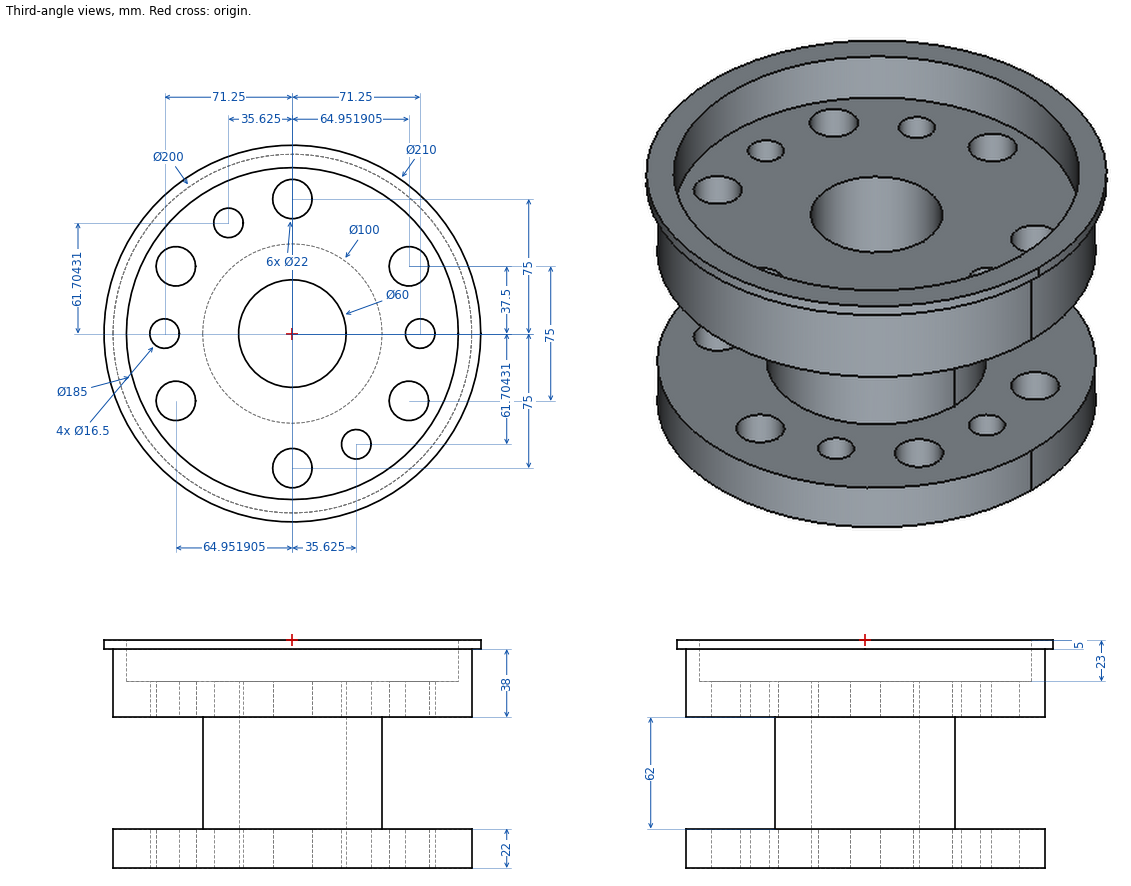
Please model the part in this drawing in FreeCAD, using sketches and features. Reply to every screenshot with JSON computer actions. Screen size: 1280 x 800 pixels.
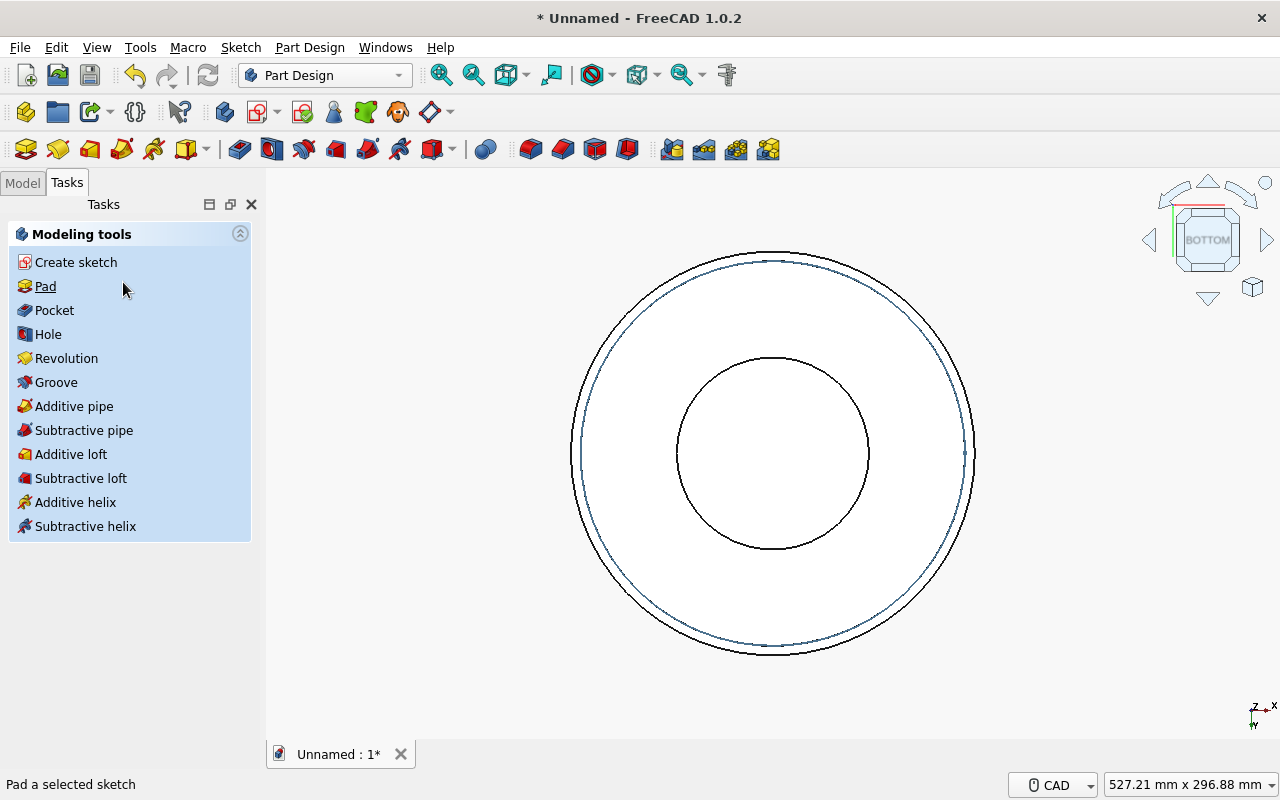
{"action": "left_click", "coordinate": [26, 150]}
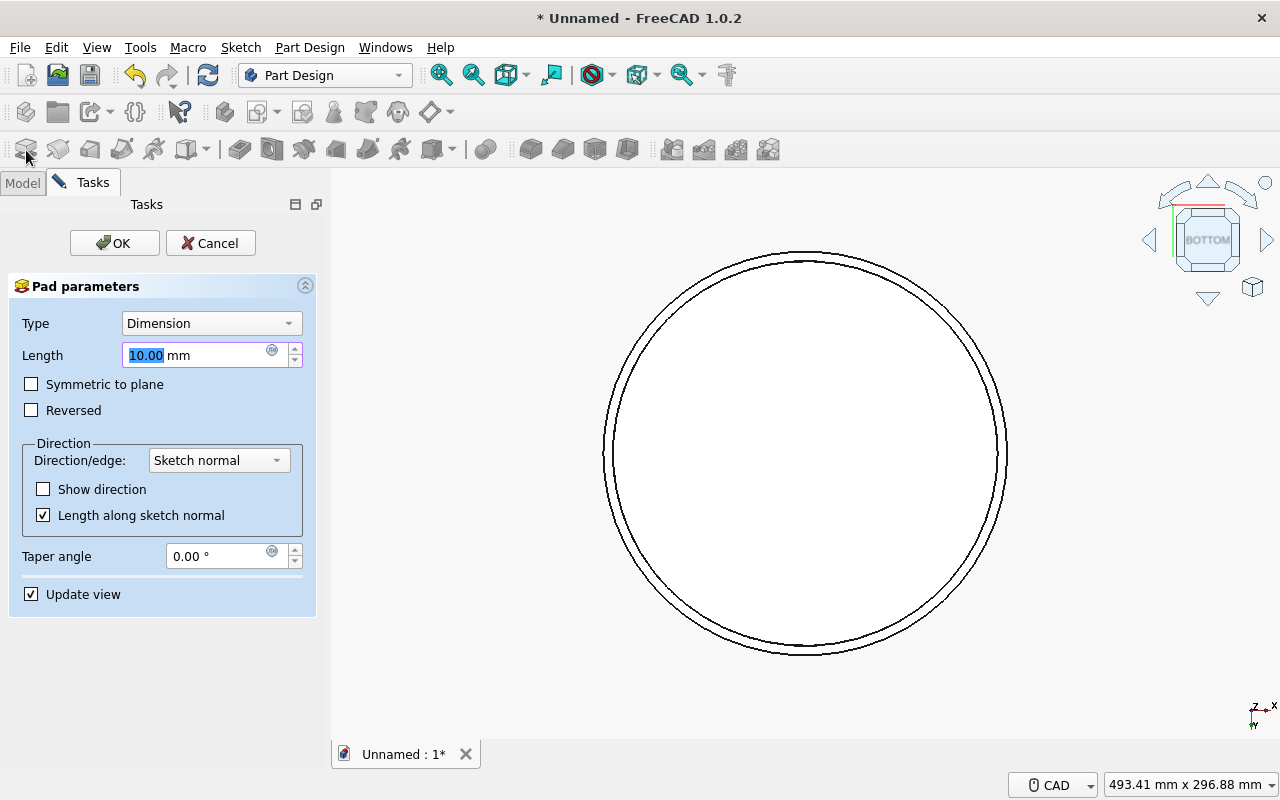
{"action": "type", "text": "22"}
{"action": "key", "text": "Tab"}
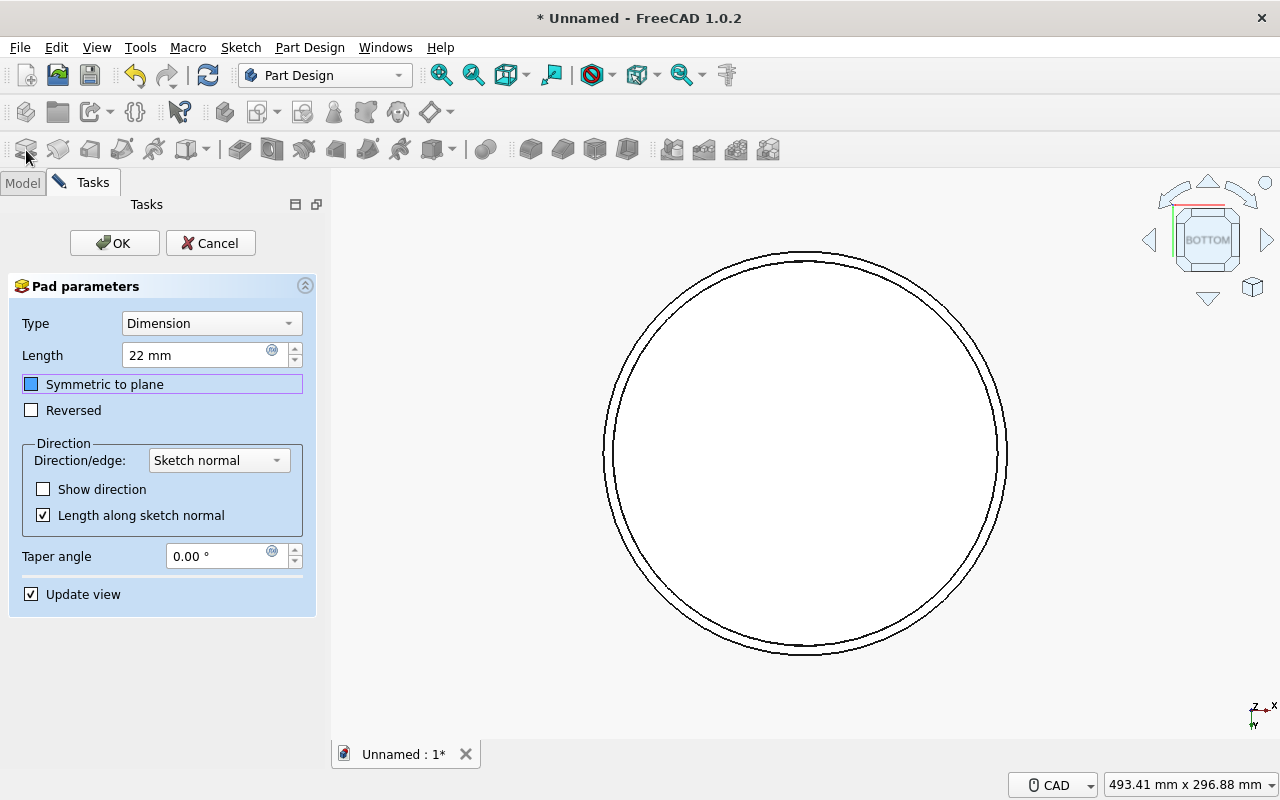
{"action": "left_click", "coordinate": [115, 243]}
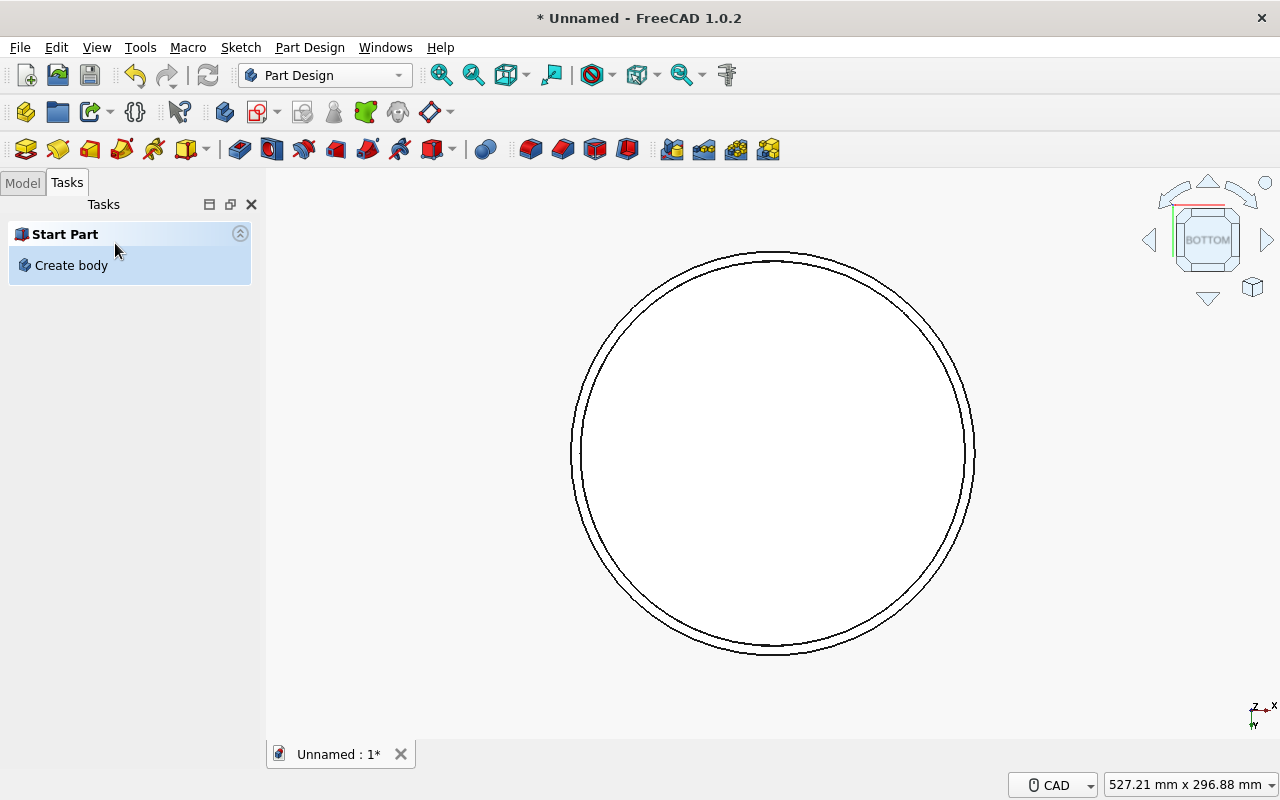
{"action": "key", "text": "0"}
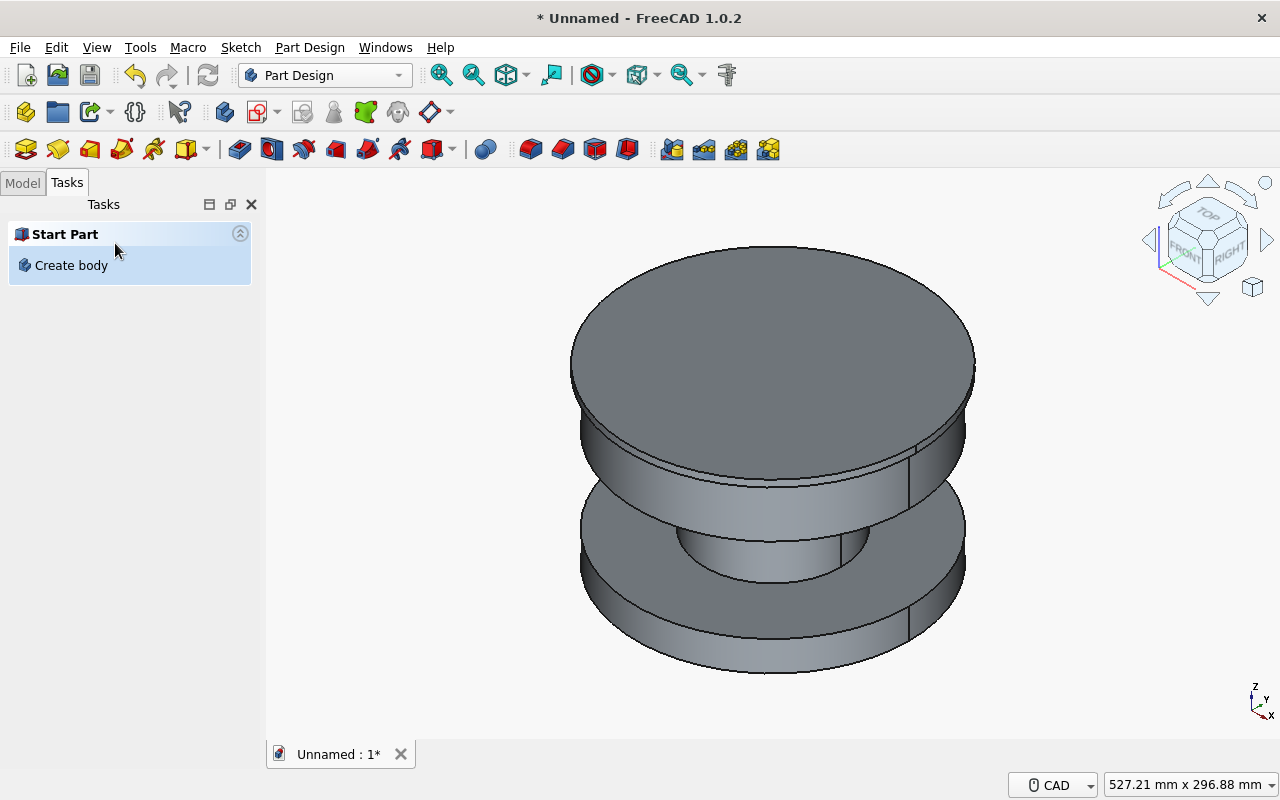
{"action": "left_click", "coordinate": [773, 362]}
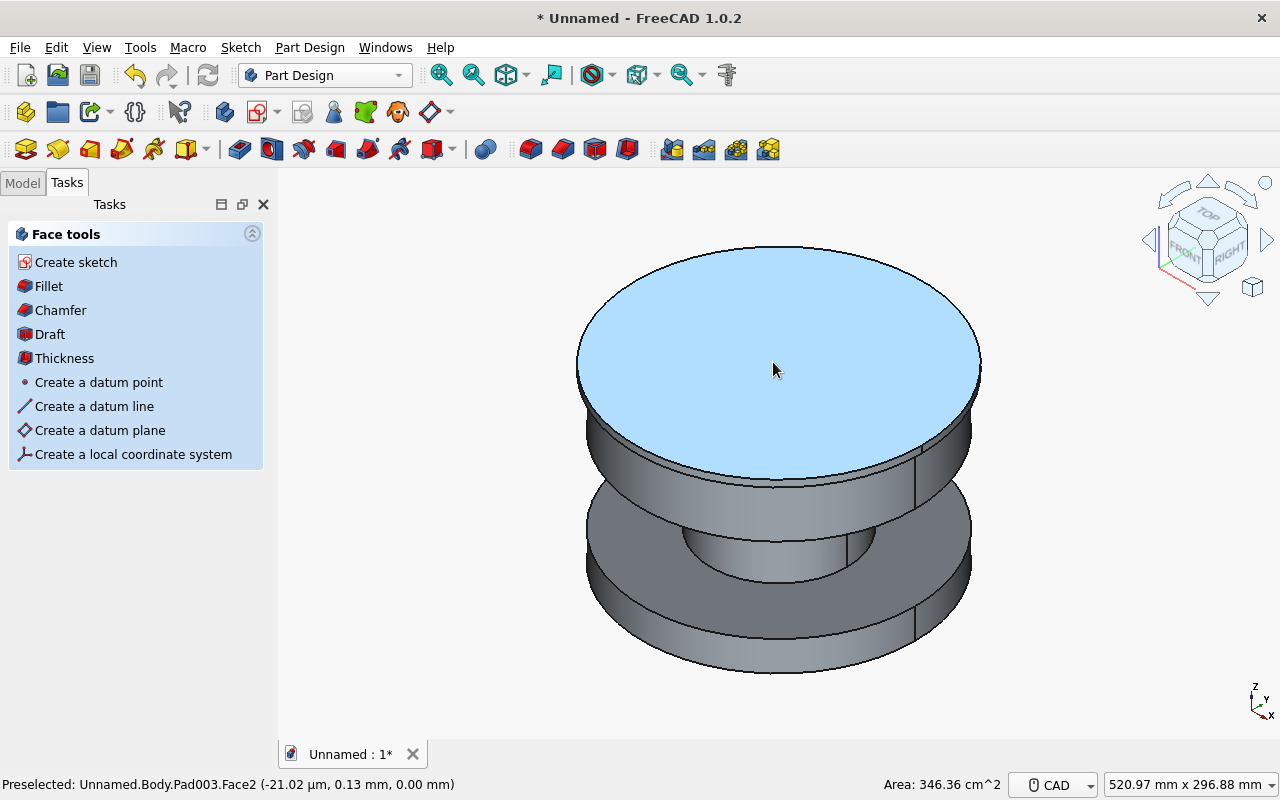
{"action": "left_click", "coordinate": [258, 112]}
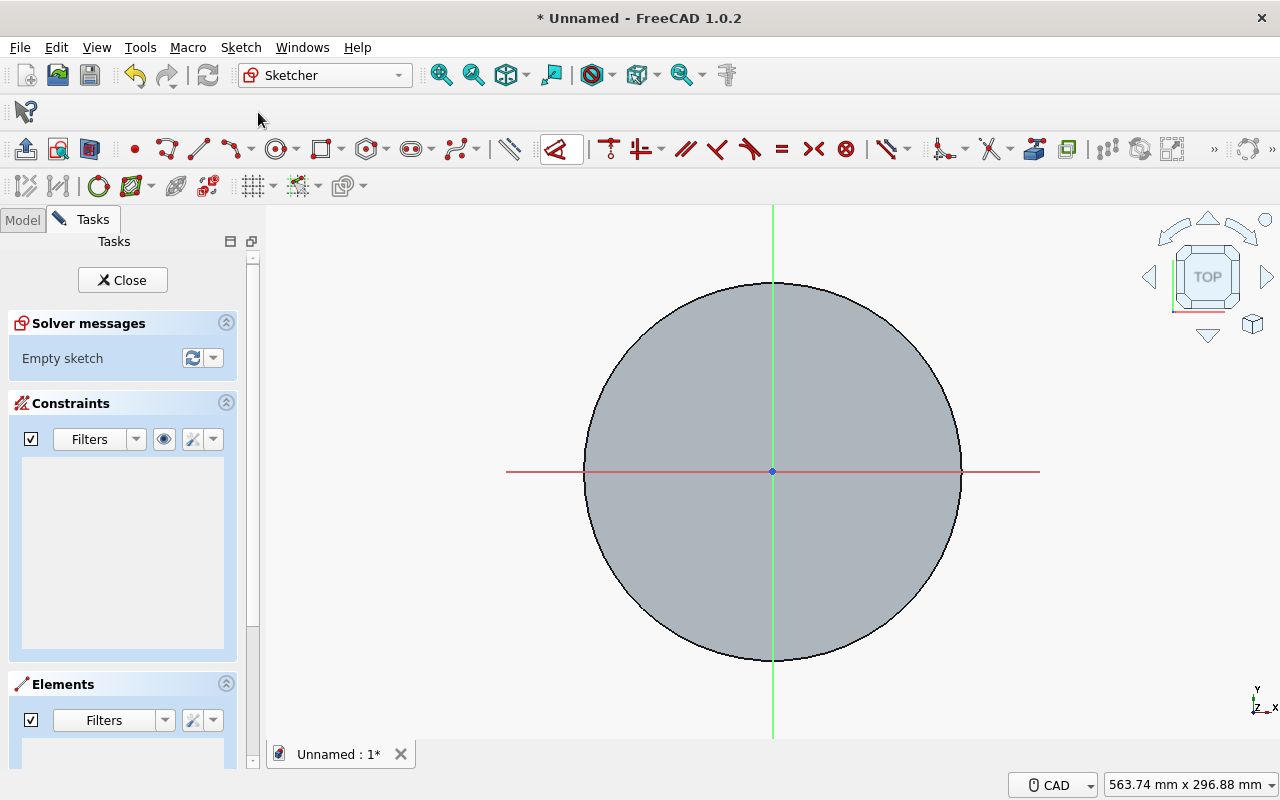
{"action": "left_click", "coordinate": [276, 150]}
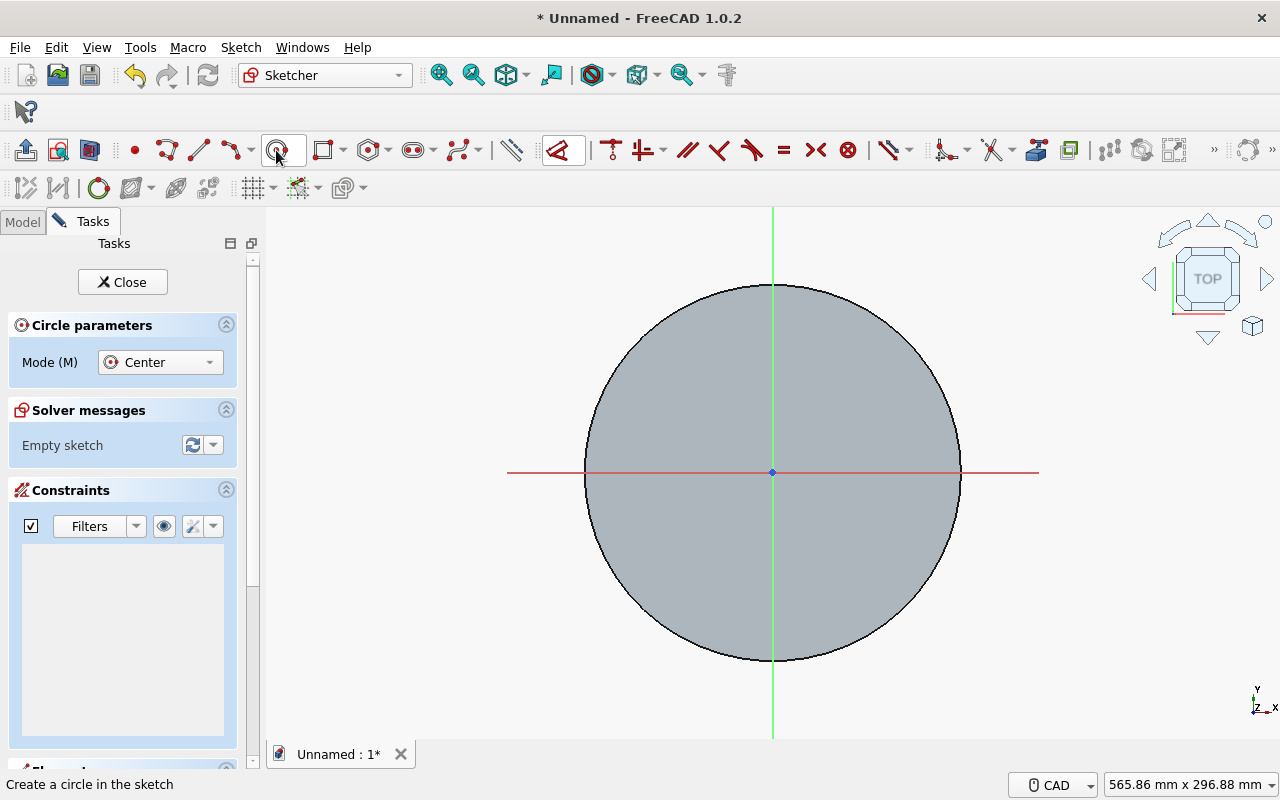
{"action": "left_click", "coordinate": [773, 473]}
{"action": "mouse_move", "coordinate": [890, 356]}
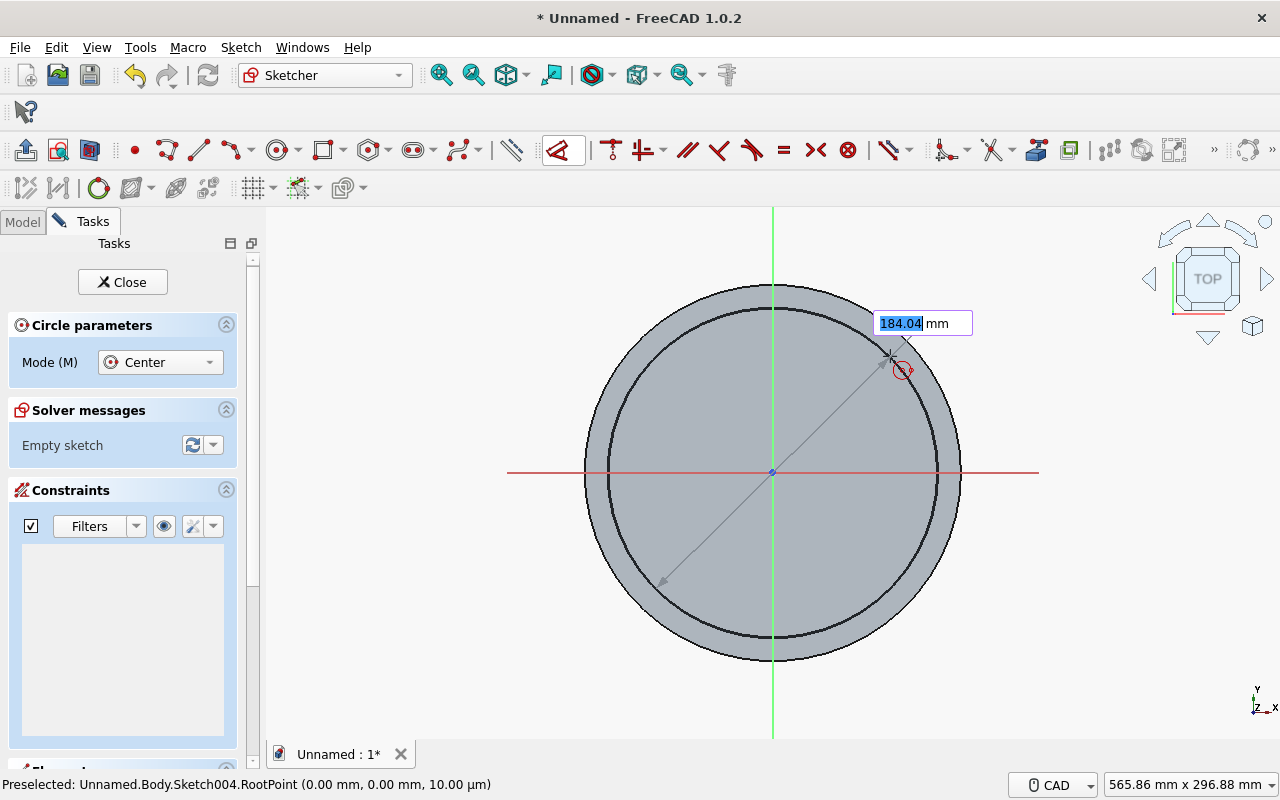
{"action": "type", "text": "185"}
{"action": "key", "text": "Return"}
{"action": "key", "text": "Escape"}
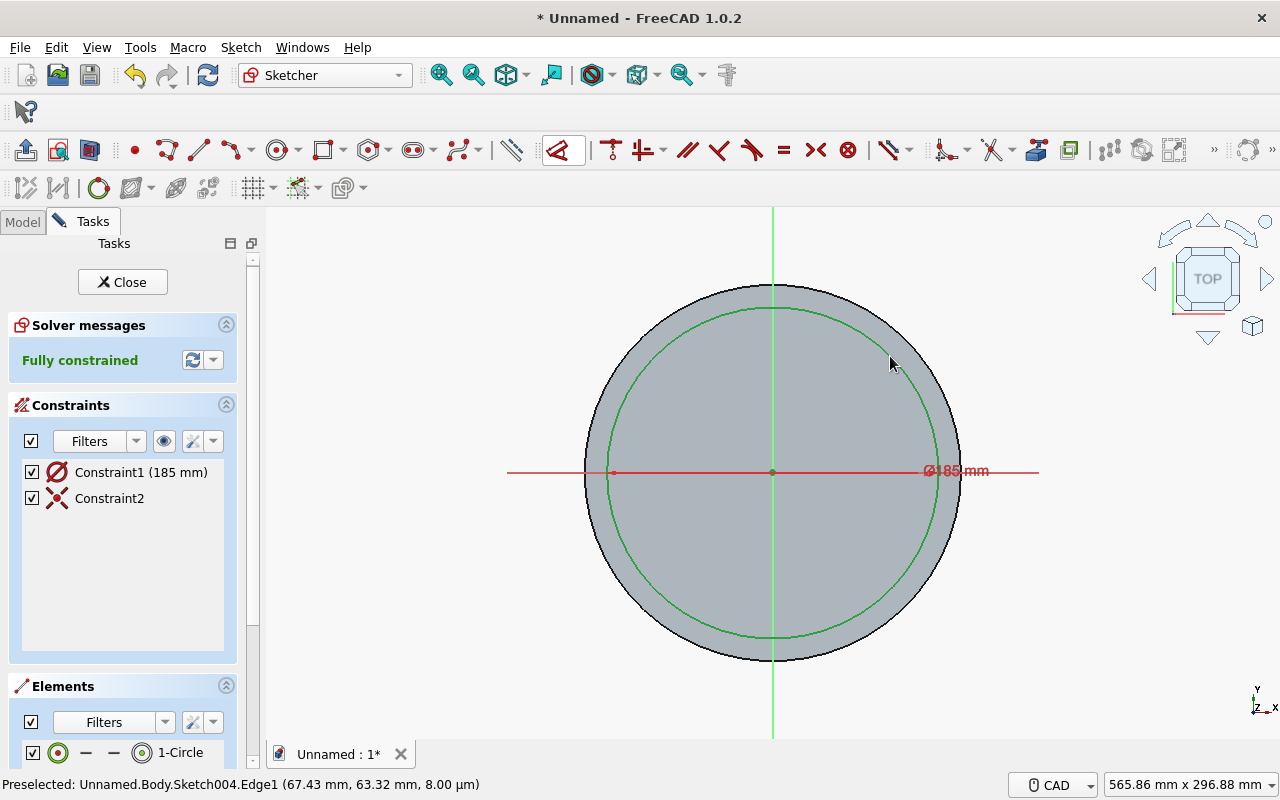
{"action": "left_click", "coordinate": [123, 282]}